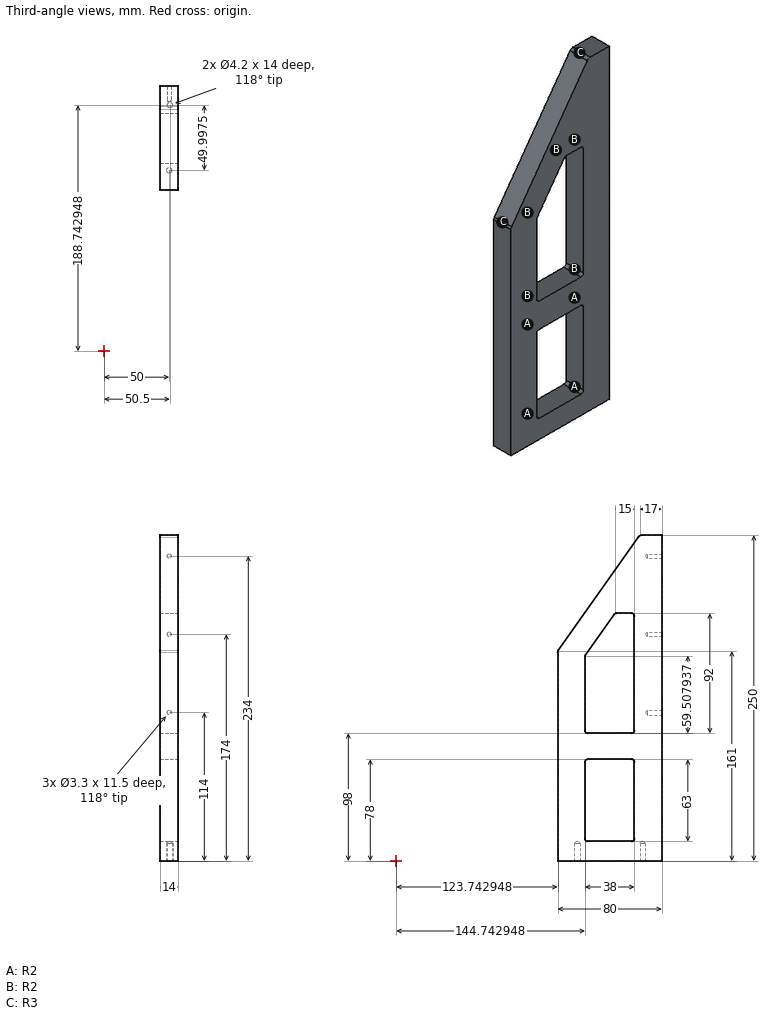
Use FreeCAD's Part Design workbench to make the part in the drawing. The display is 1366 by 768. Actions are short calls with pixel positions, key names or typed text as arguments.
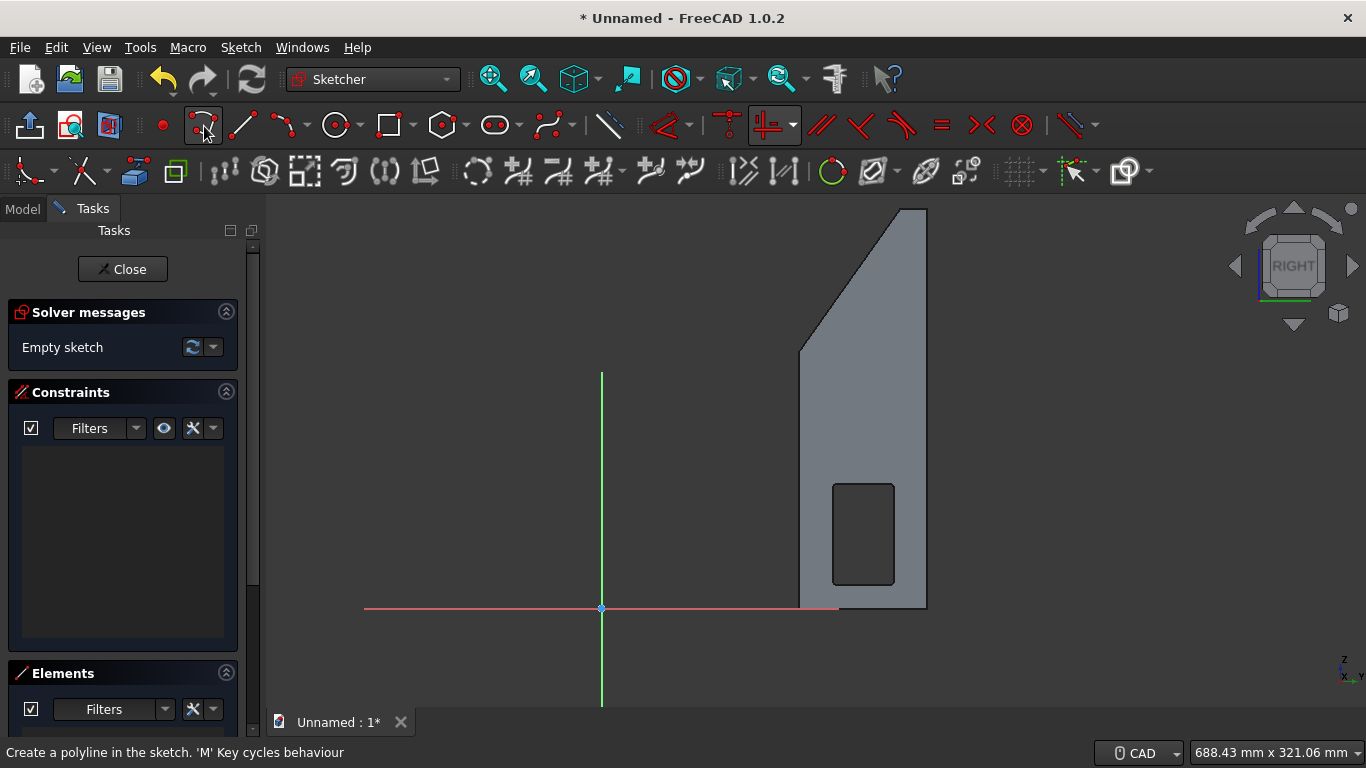
click(833, 452)
click(894, 452)
click(894, 305)
click(870, 305)
click(833, 357)
click(833, 453)
key(Escape)
key(Escape)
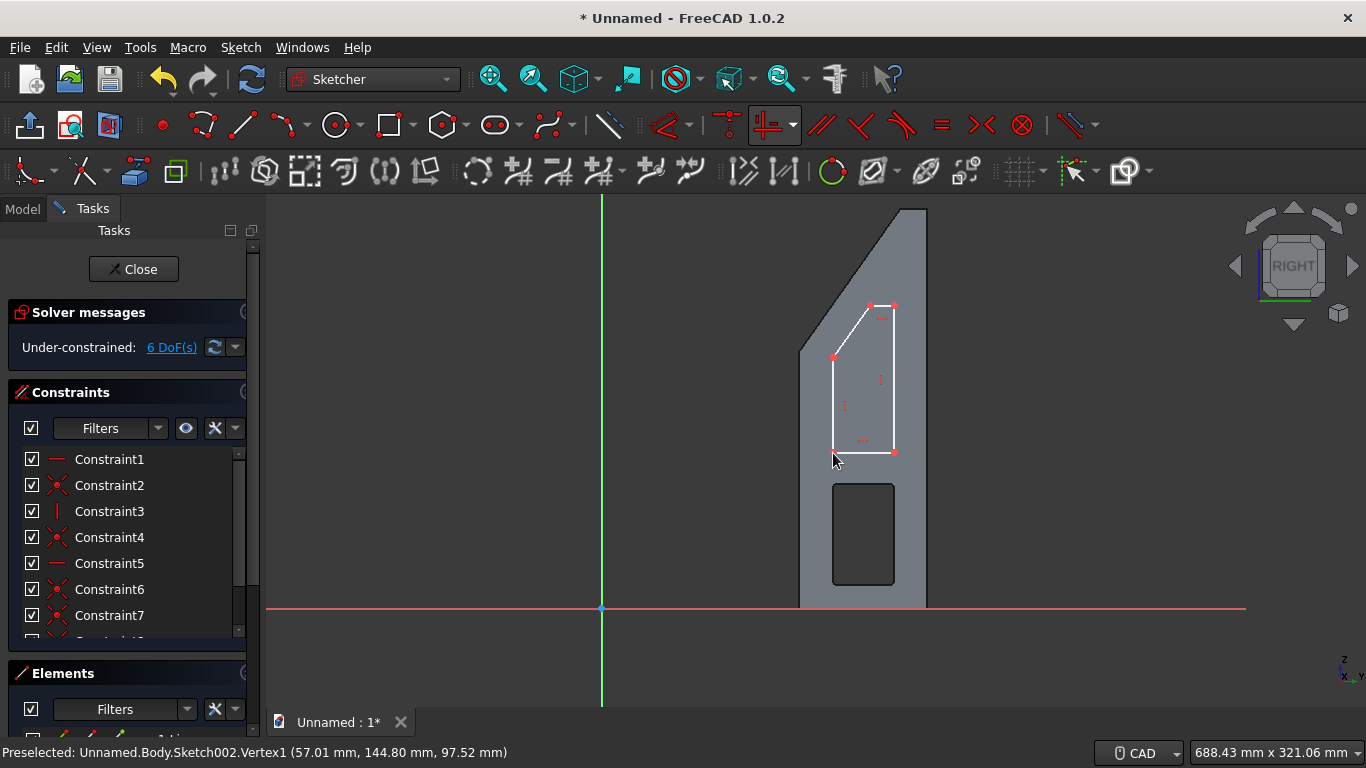
click(664, 126)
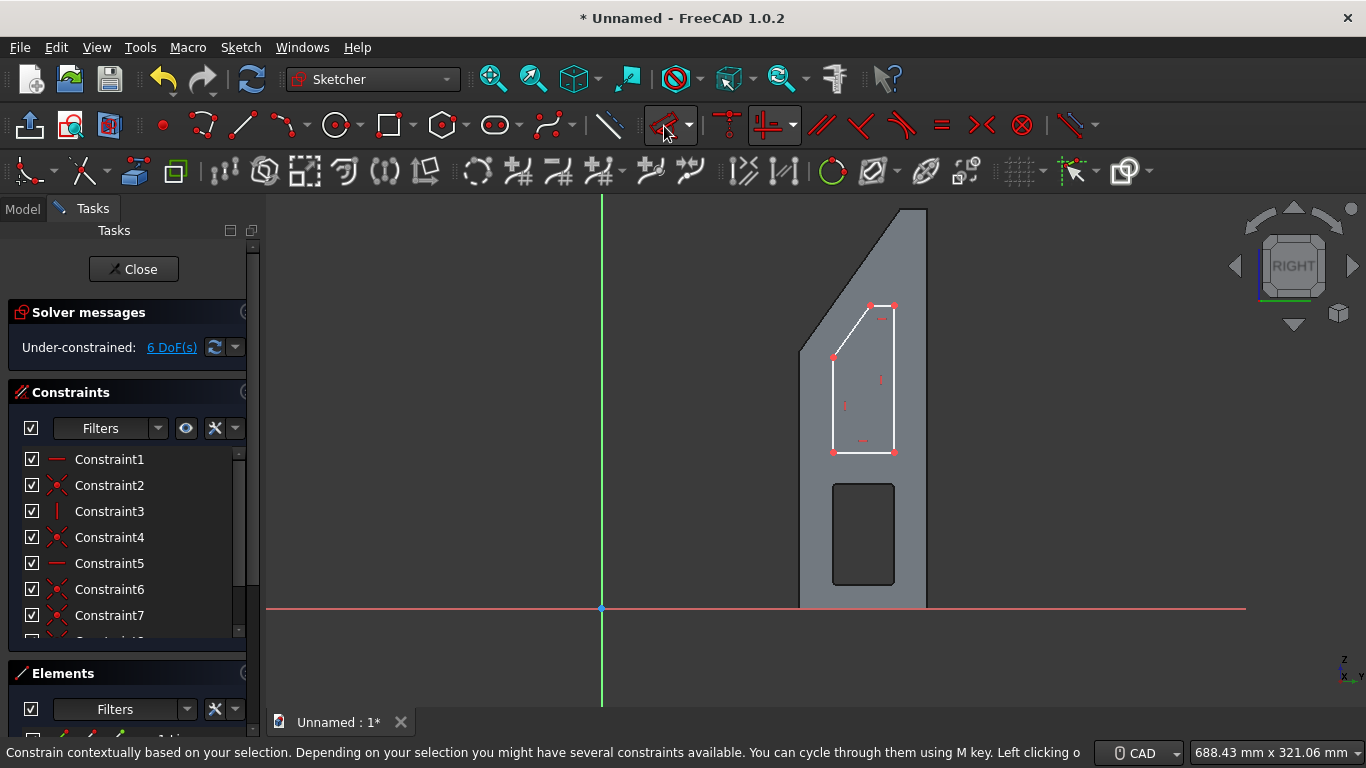
click(851, 453)
click(863, 419)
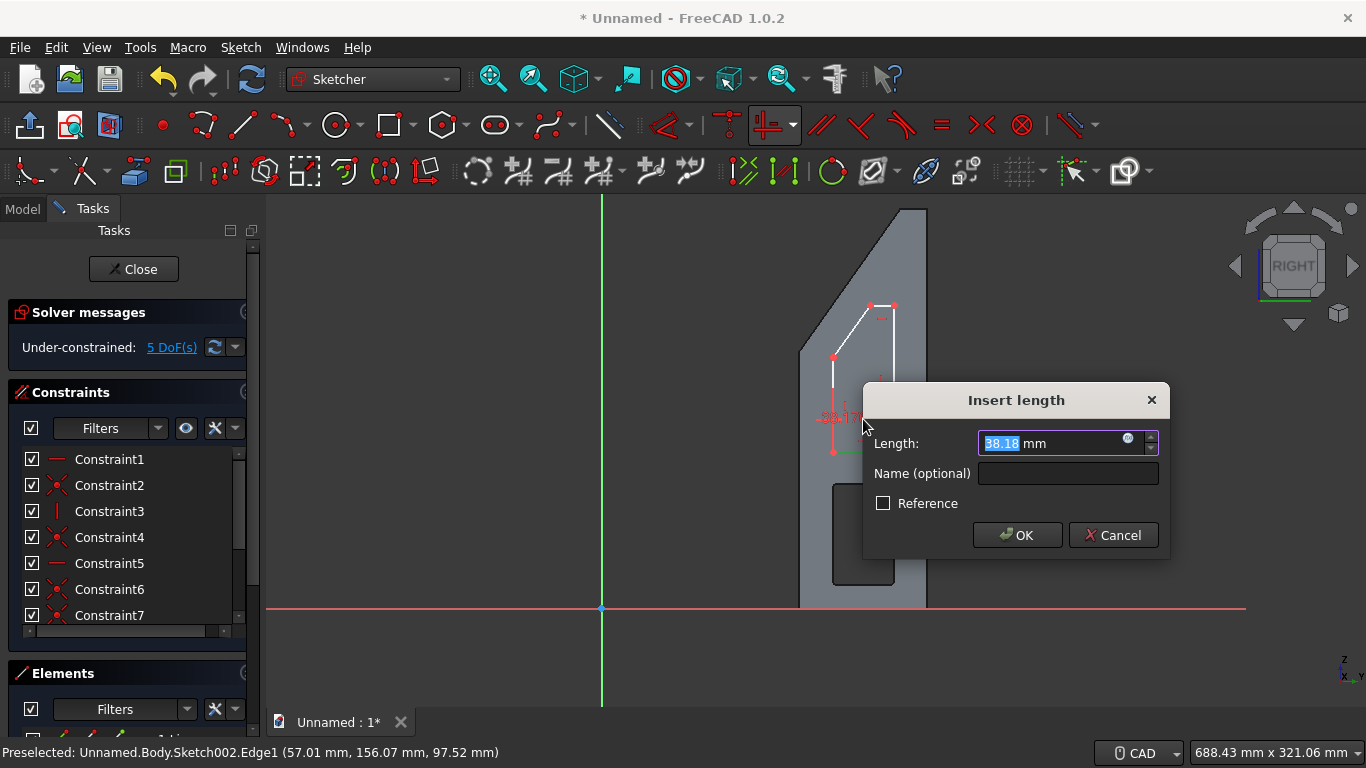
text(38)
key(Return)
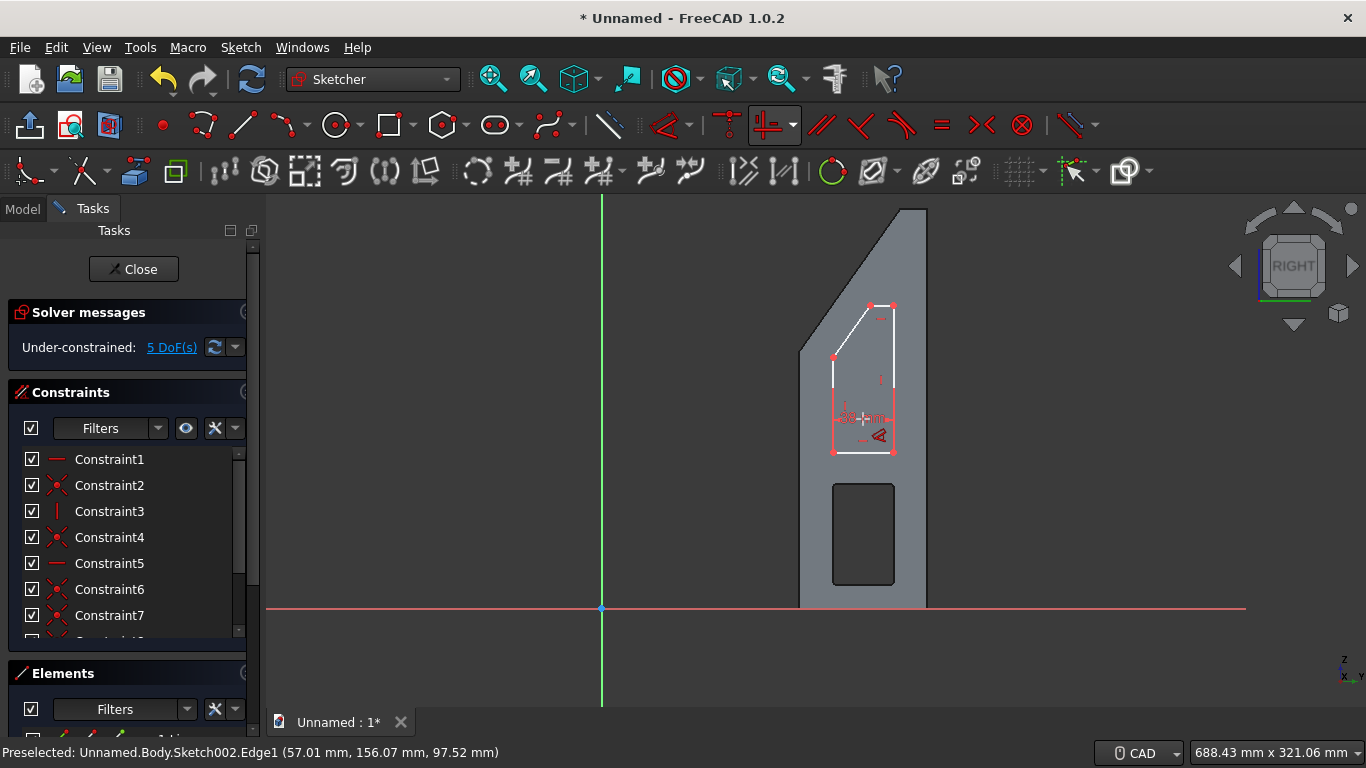
click(894, 409)
click(928, 380)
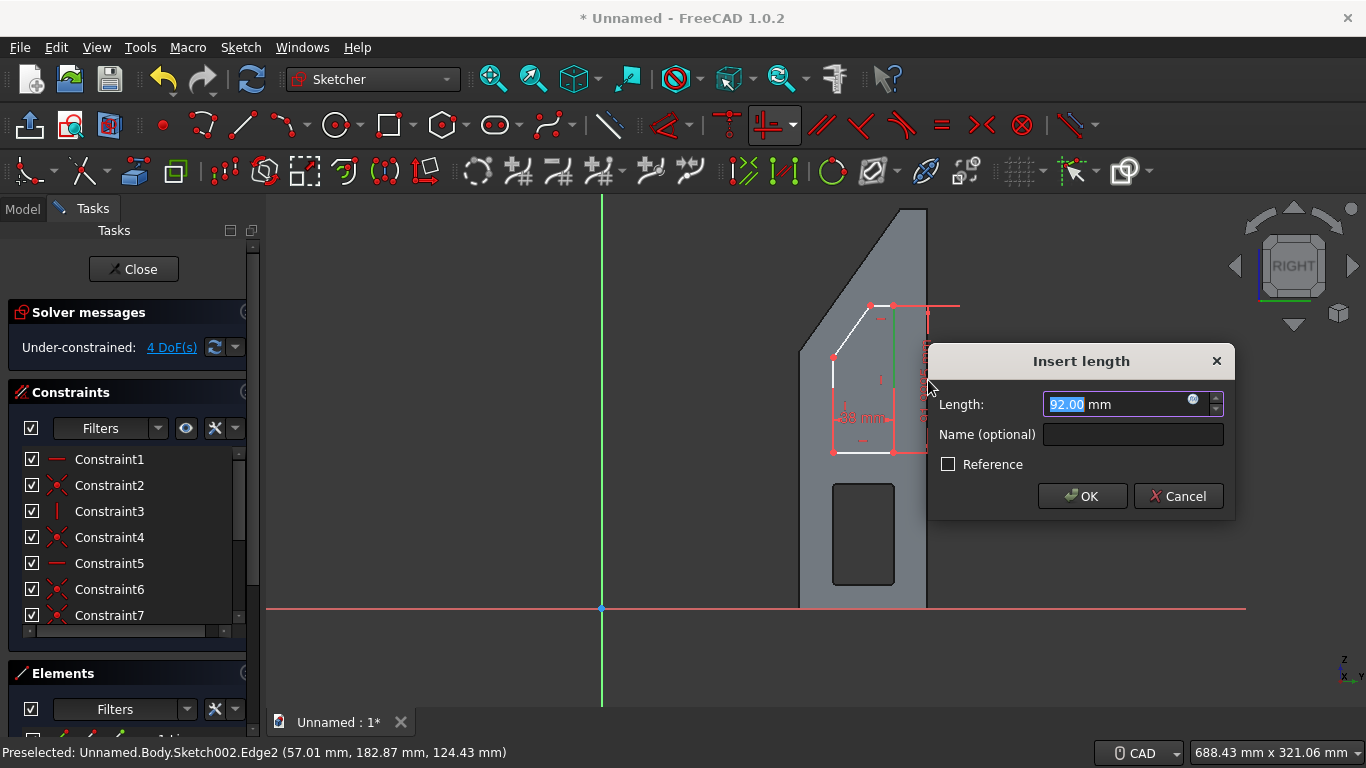
text(92)
key(Return)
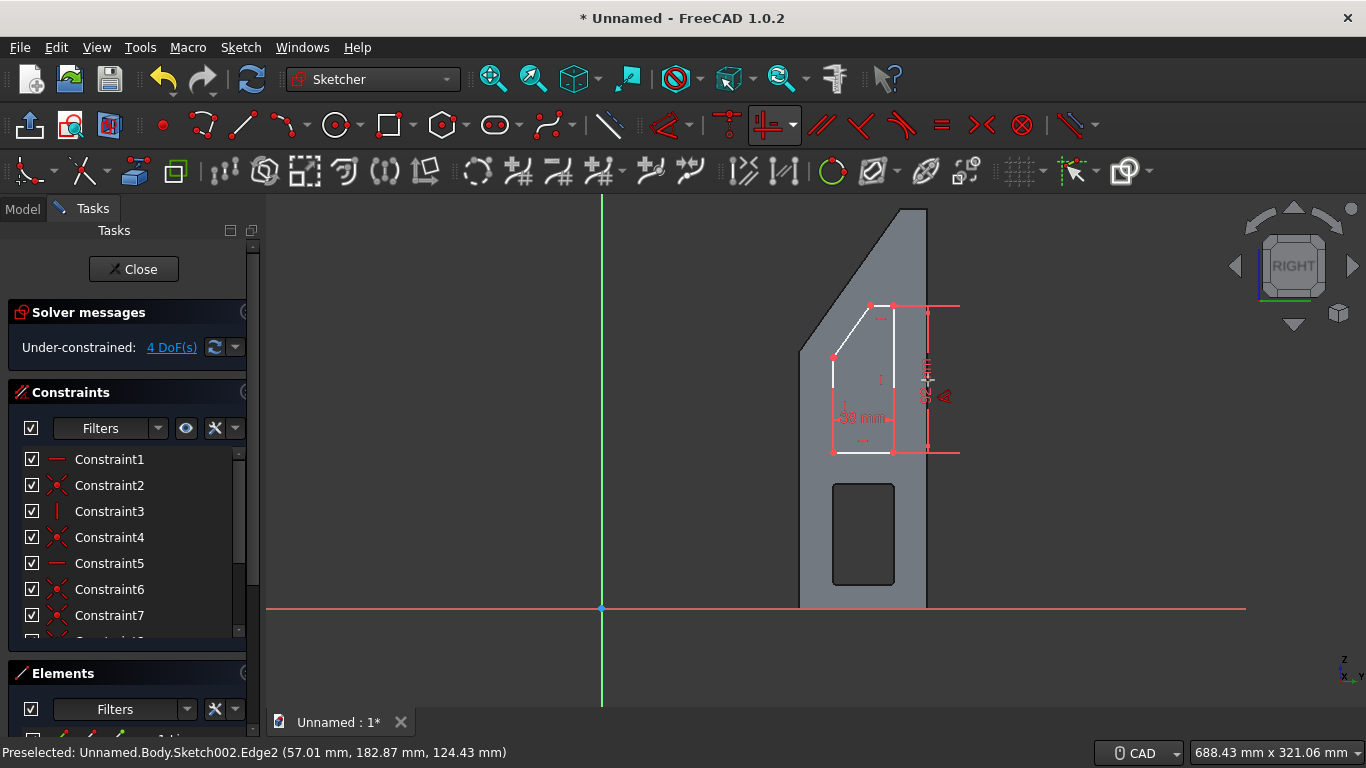
scroll(884, 306, up, 3)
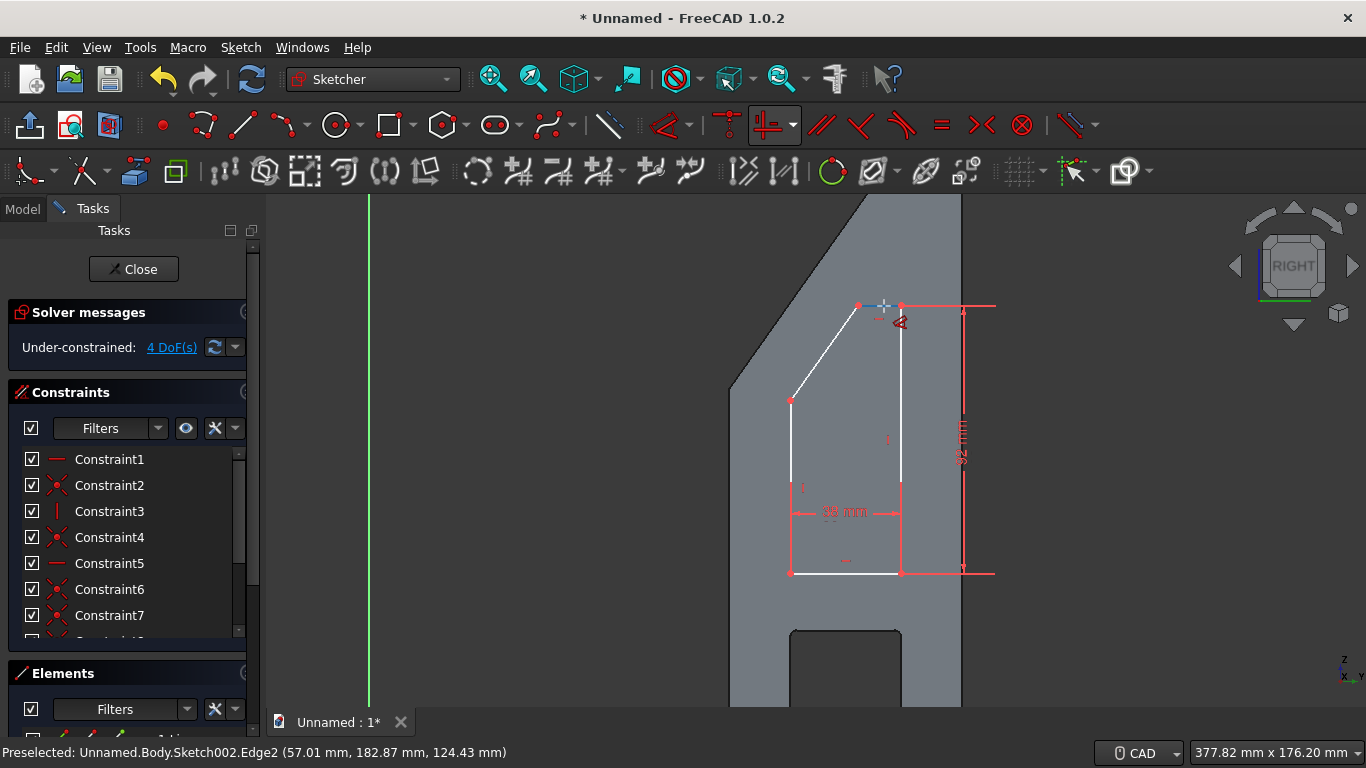
click(884, 306)
click(880, 272)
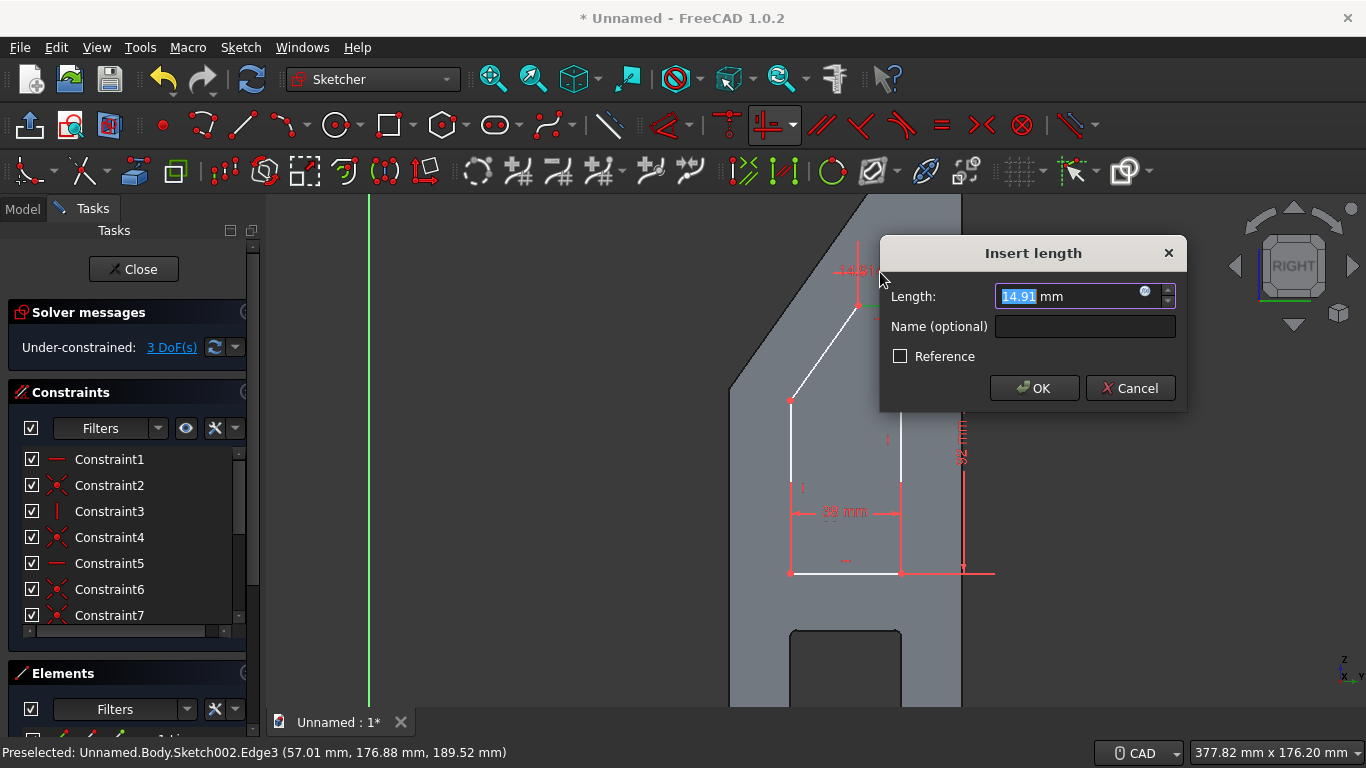
text(15)
key(Return)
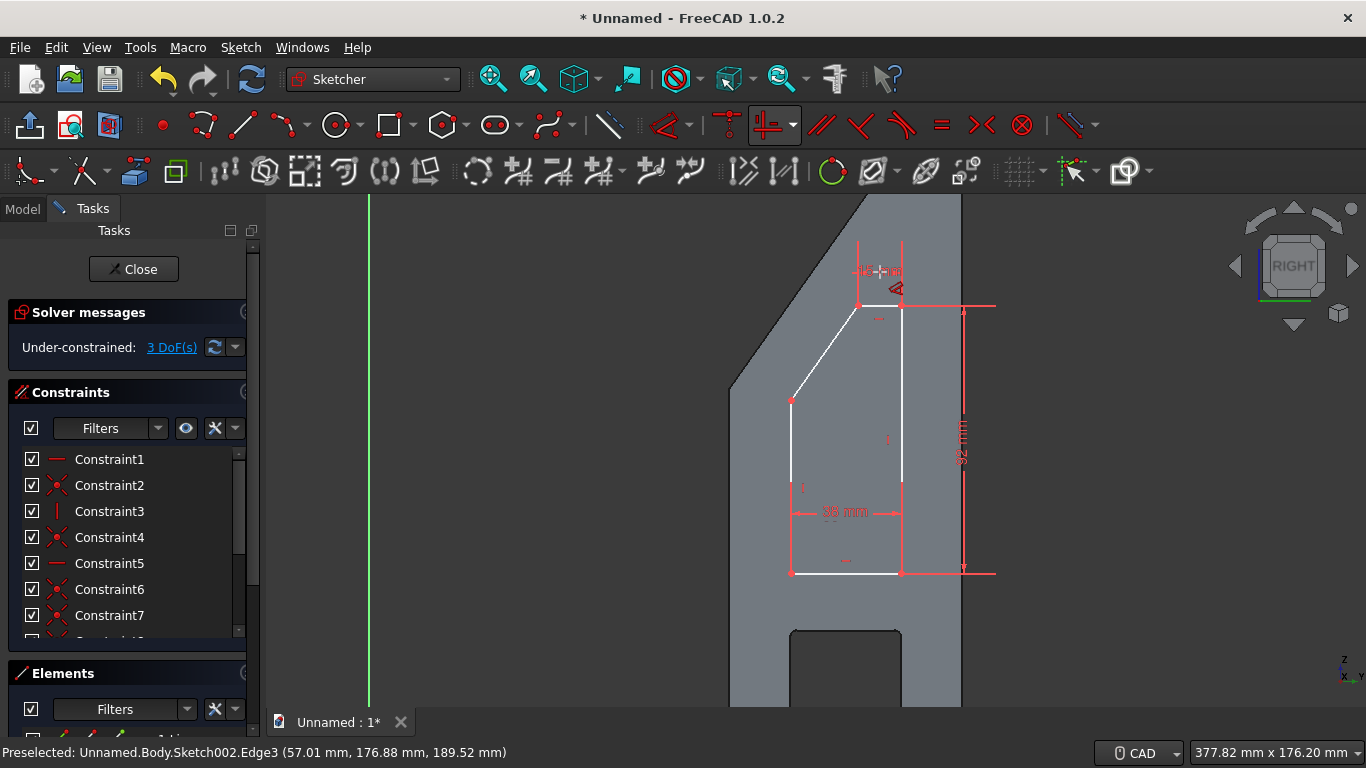
click(791, 574)
click(335, 626)